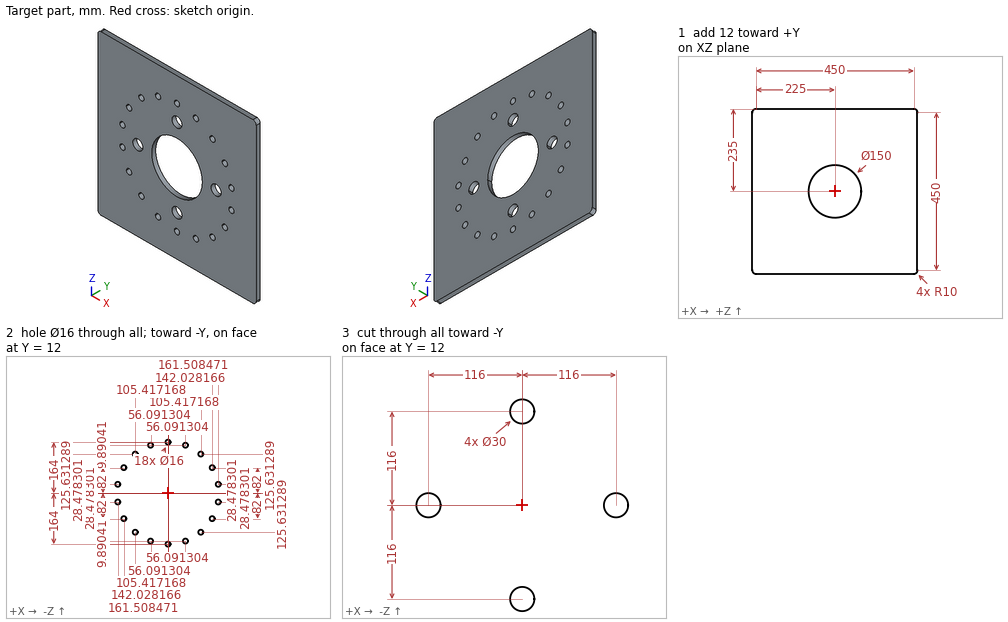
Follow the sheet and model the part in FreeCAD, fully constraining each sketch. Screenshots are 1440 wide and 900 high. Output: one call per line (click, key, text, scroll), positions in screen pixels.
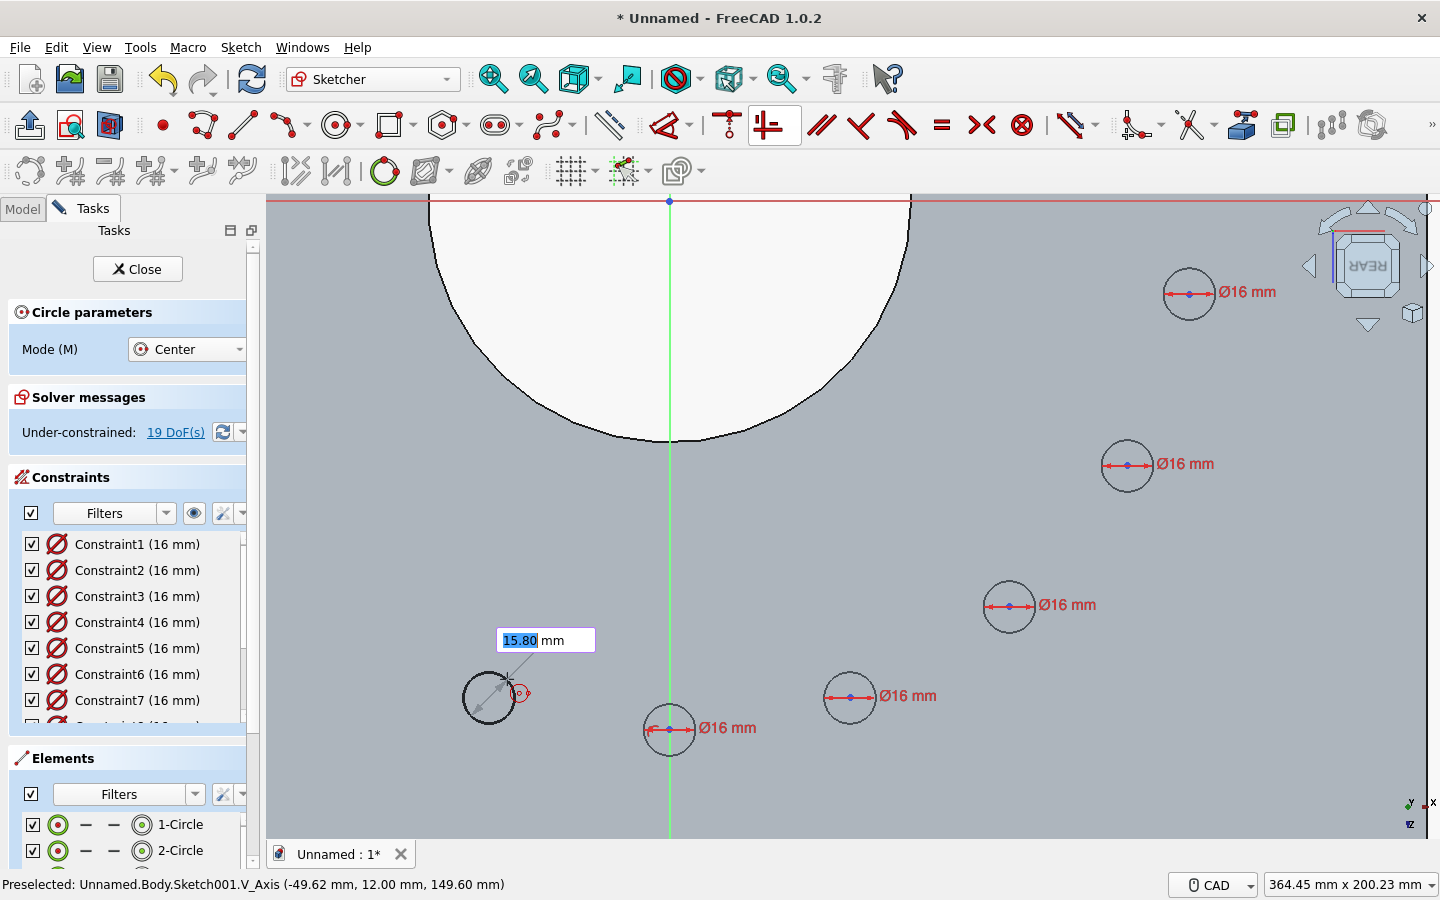
text(16)
key(Return)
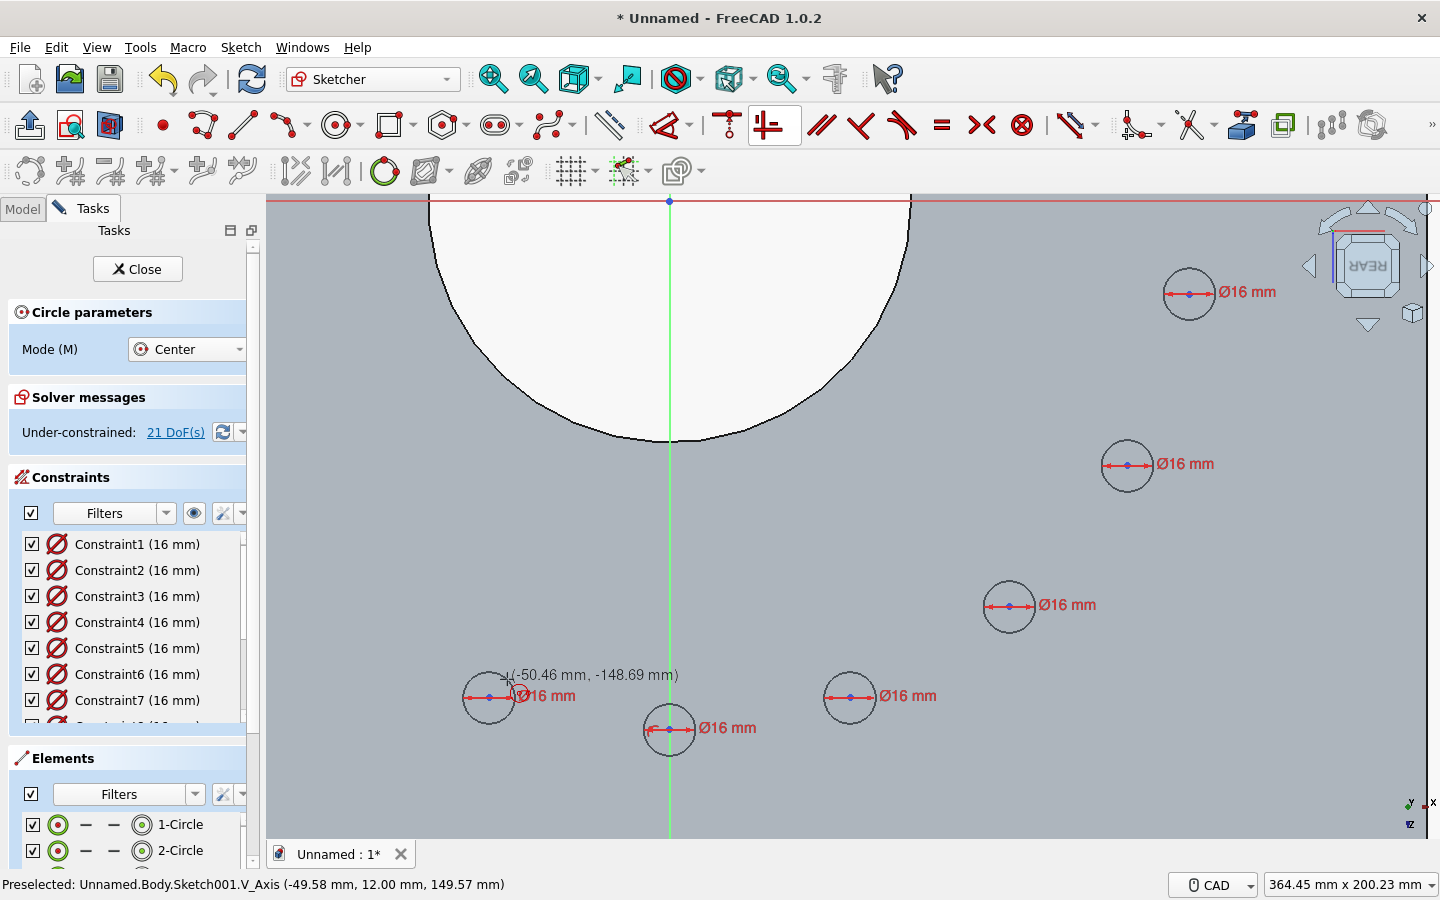
click(330, 606)
move(348, 588)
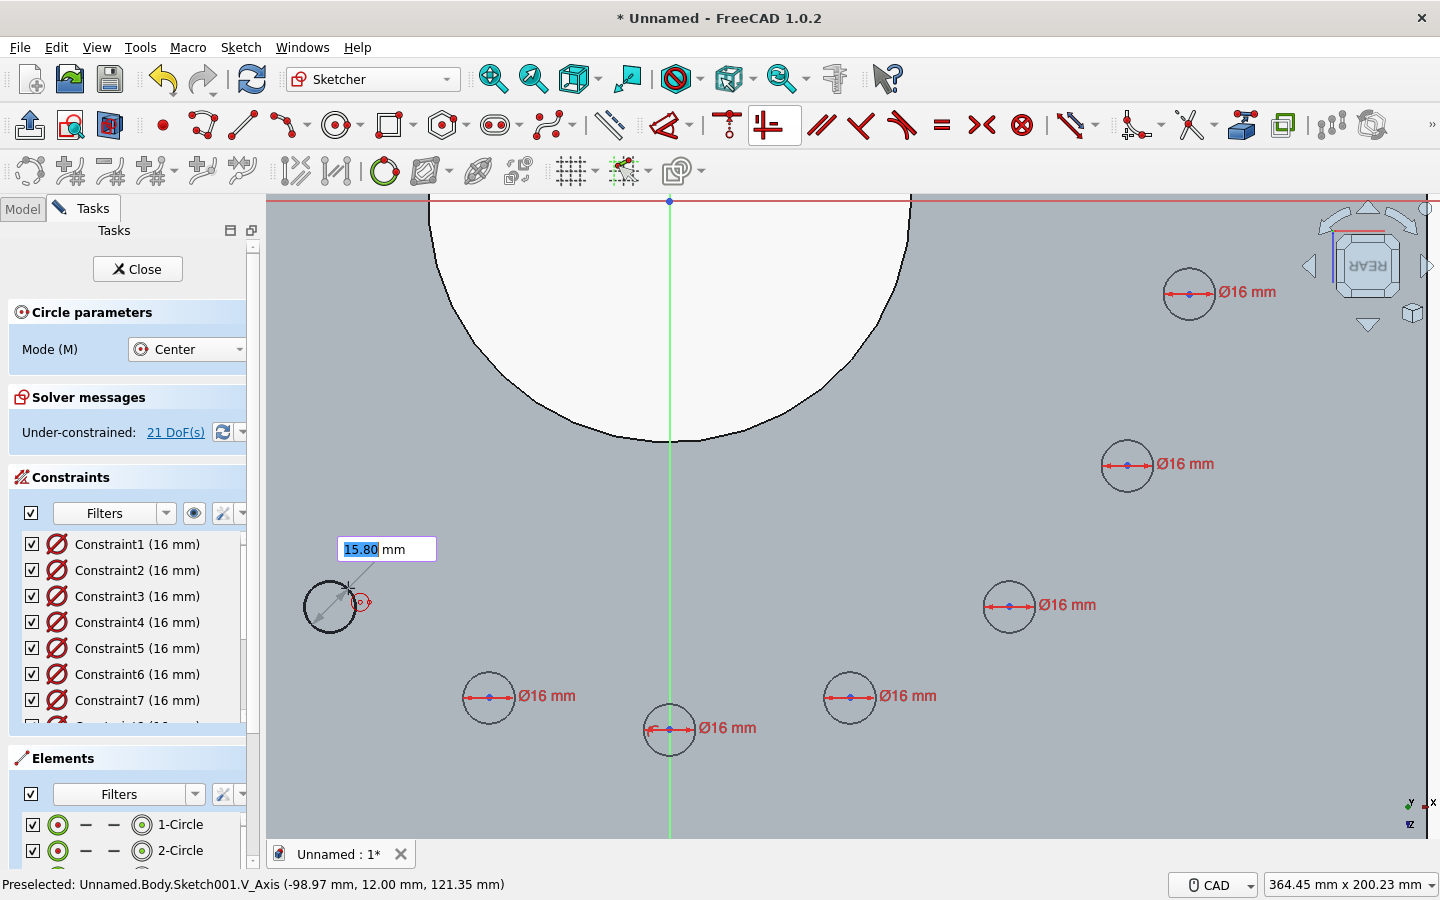
text(16)
key(Return)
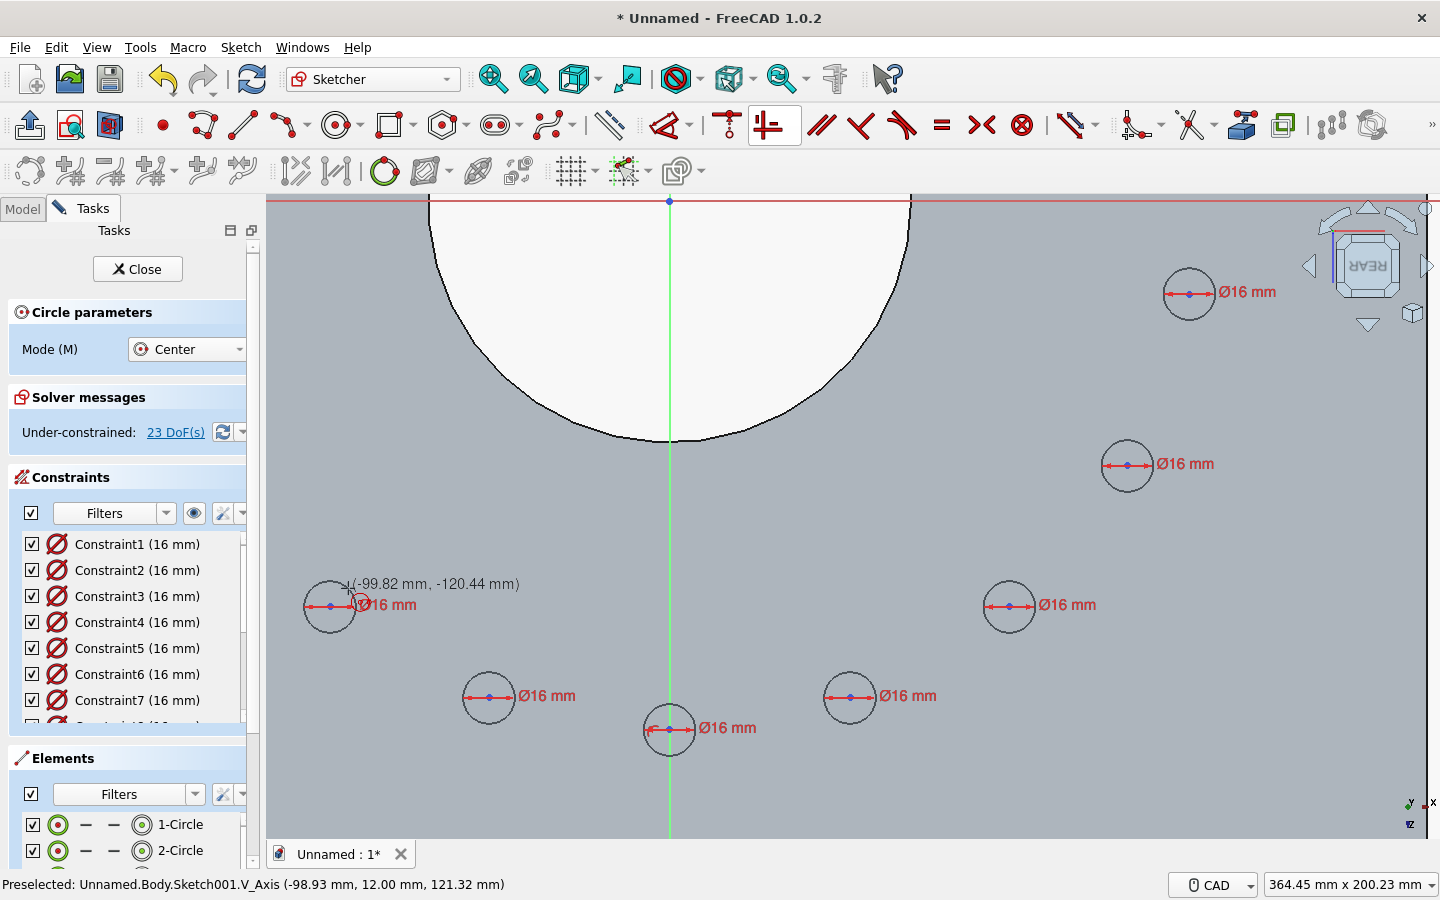
scroll(851, 700, down, 5)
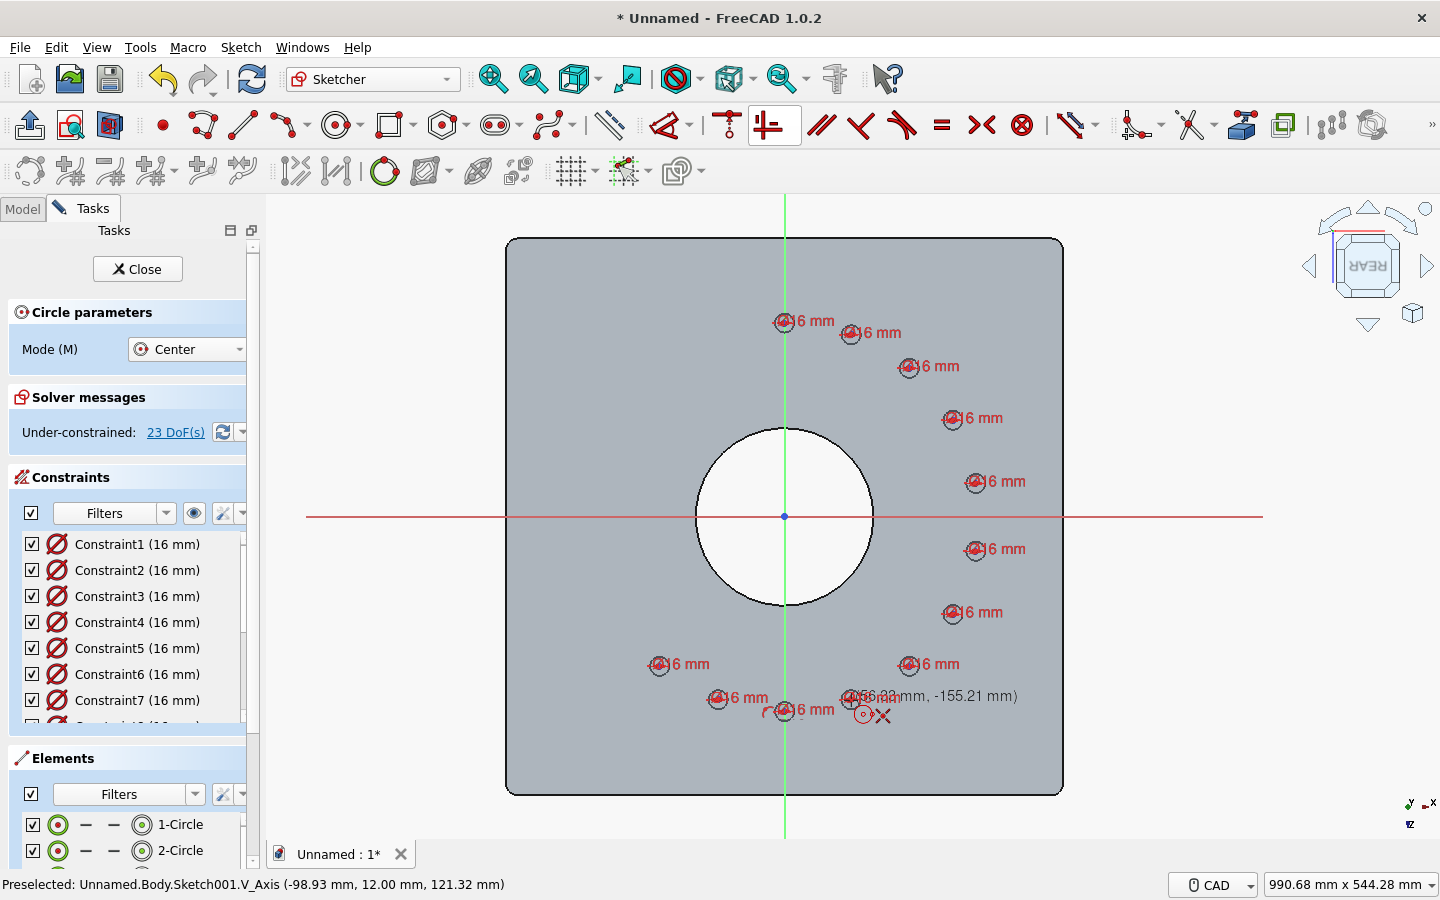
scroll(616, 614, up, 5)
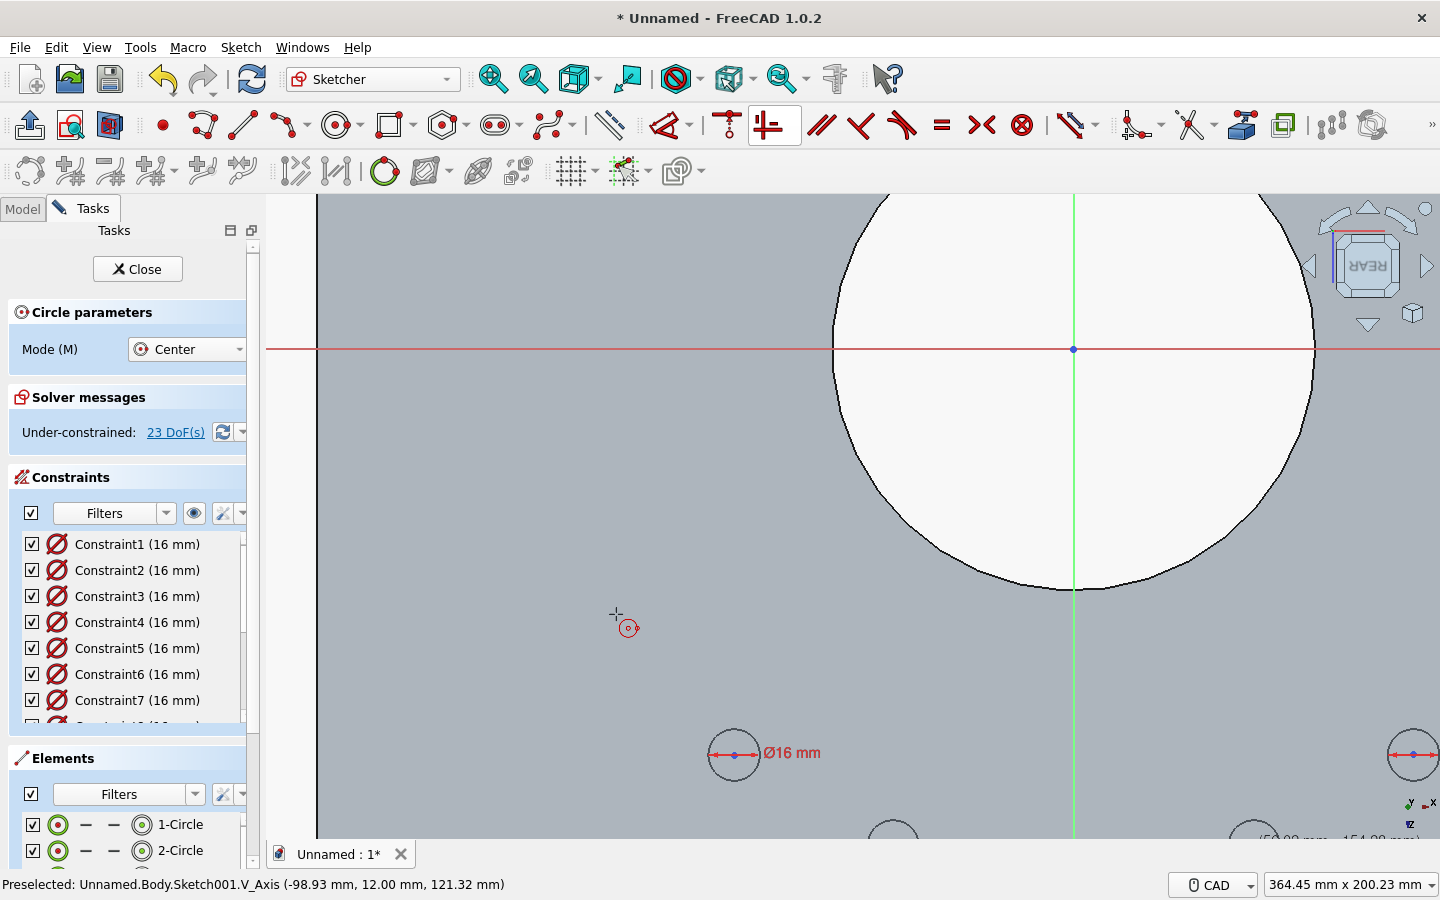
click(616, 613)
move(634, 595)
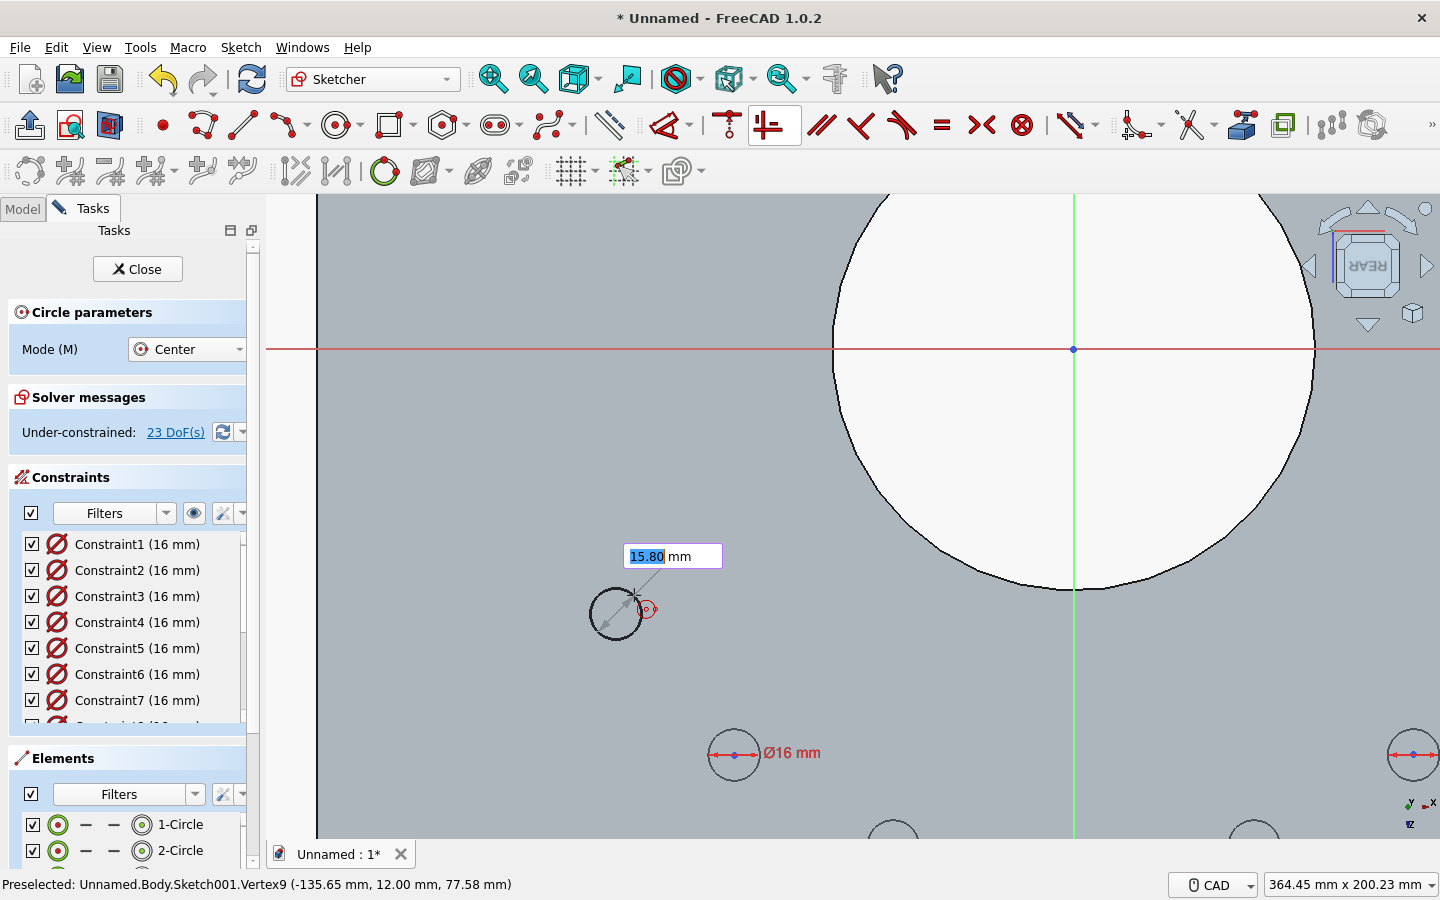
text(16)
key(Return)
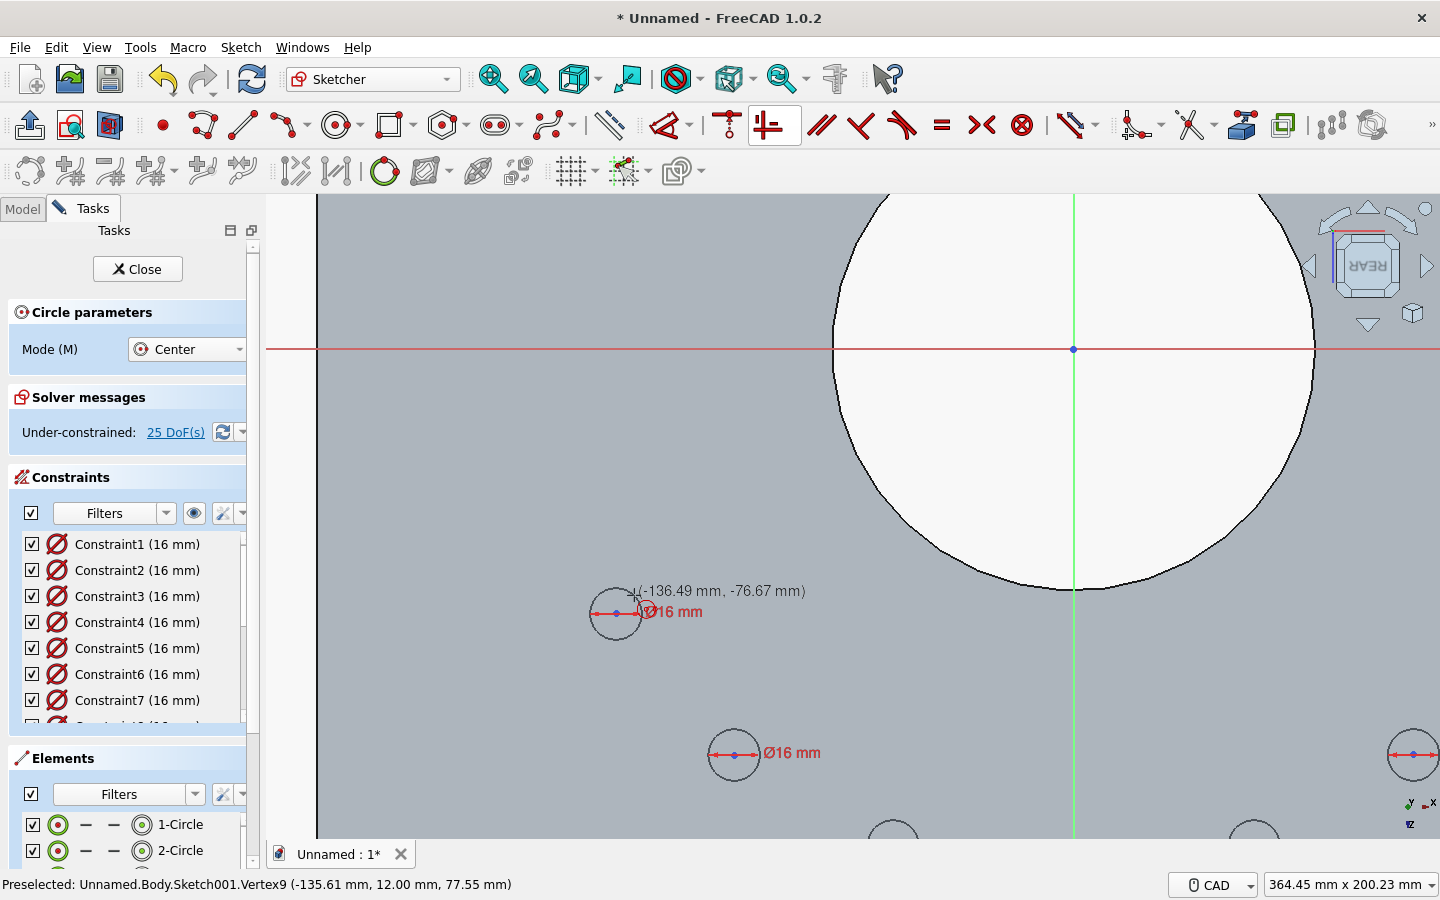
click(553, 441)
move(572, 423)